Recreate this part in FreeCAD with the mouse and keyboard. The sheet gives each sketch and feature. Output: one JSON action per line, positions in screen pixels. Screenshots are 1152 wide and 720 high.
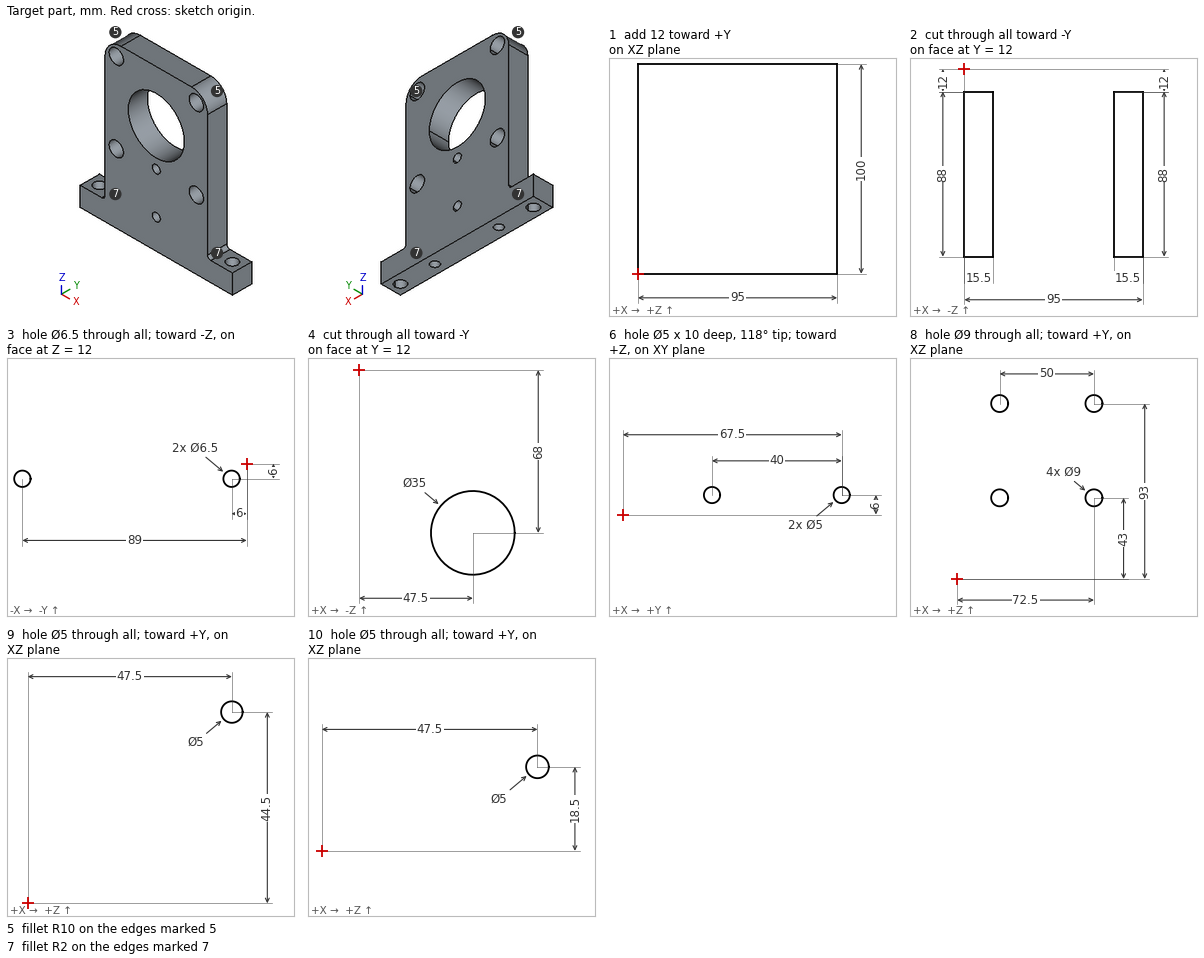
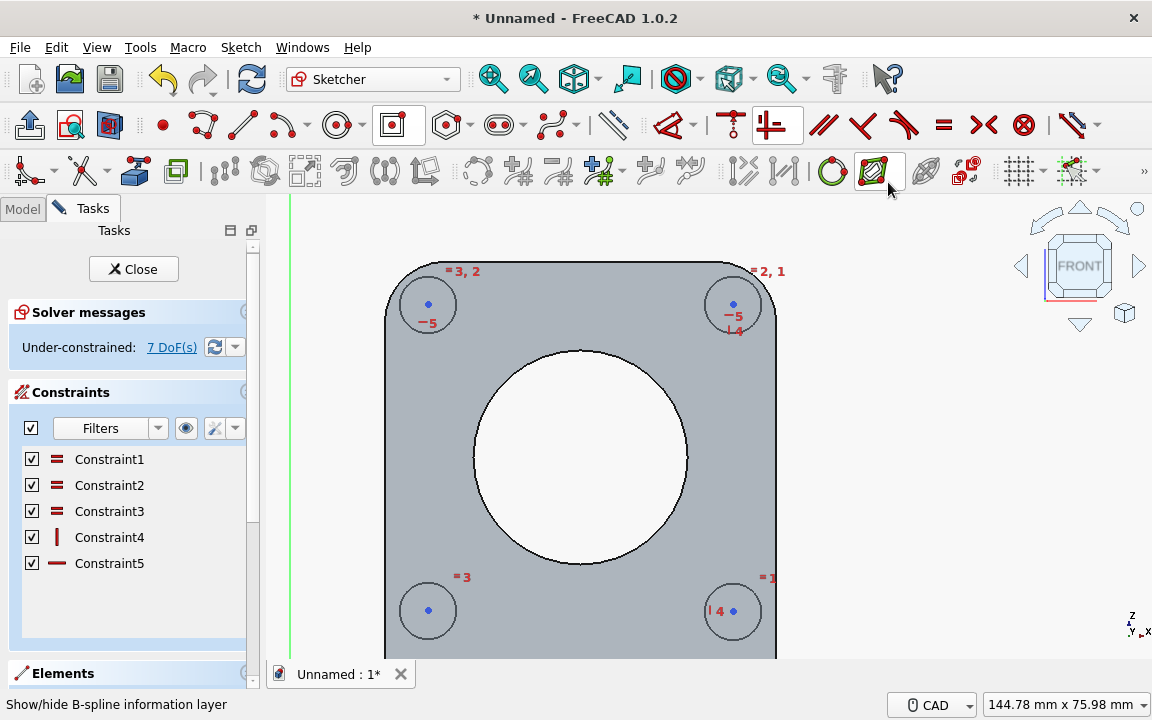
{"action": "left_click", "coordinate": [428, 305]}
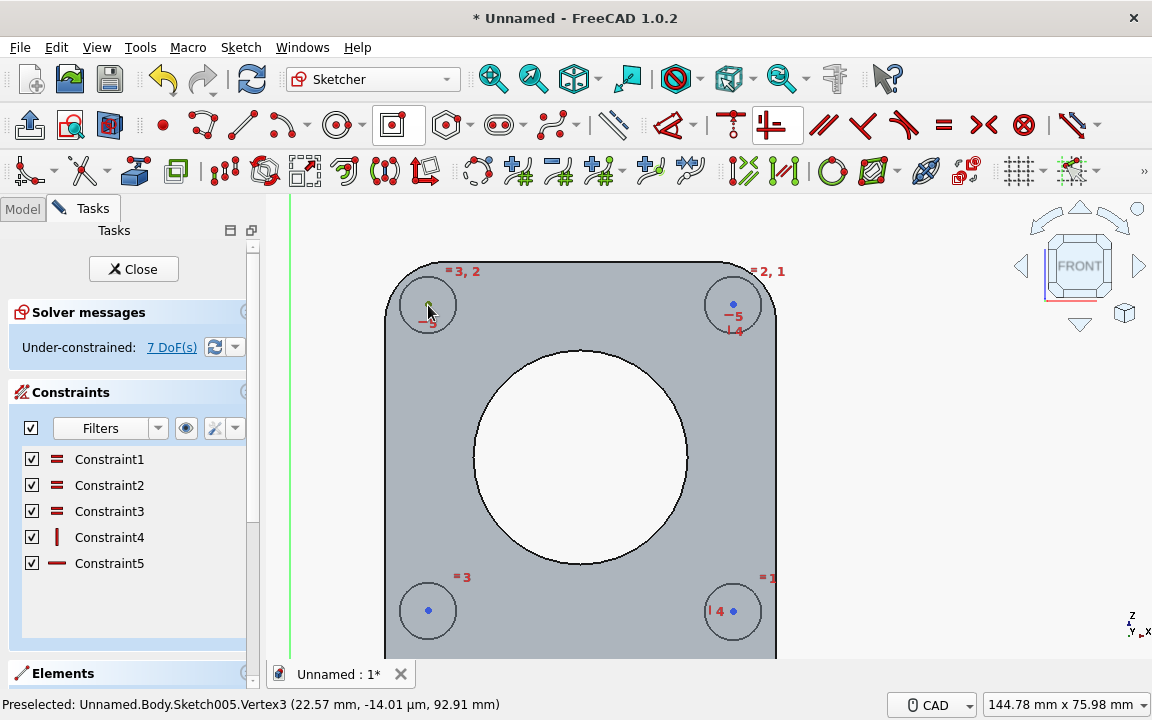
{"action": "left_click", "coordinate": [428, 611]}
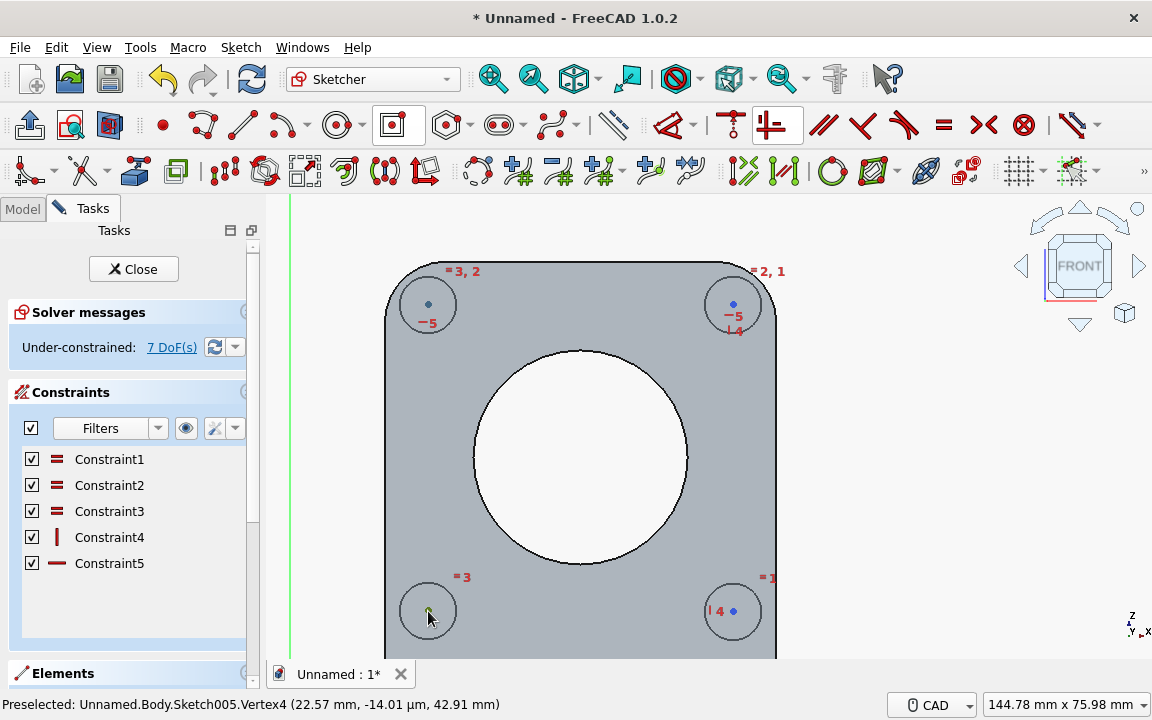
{"action": "left_click", "coordinate": [798, 126]}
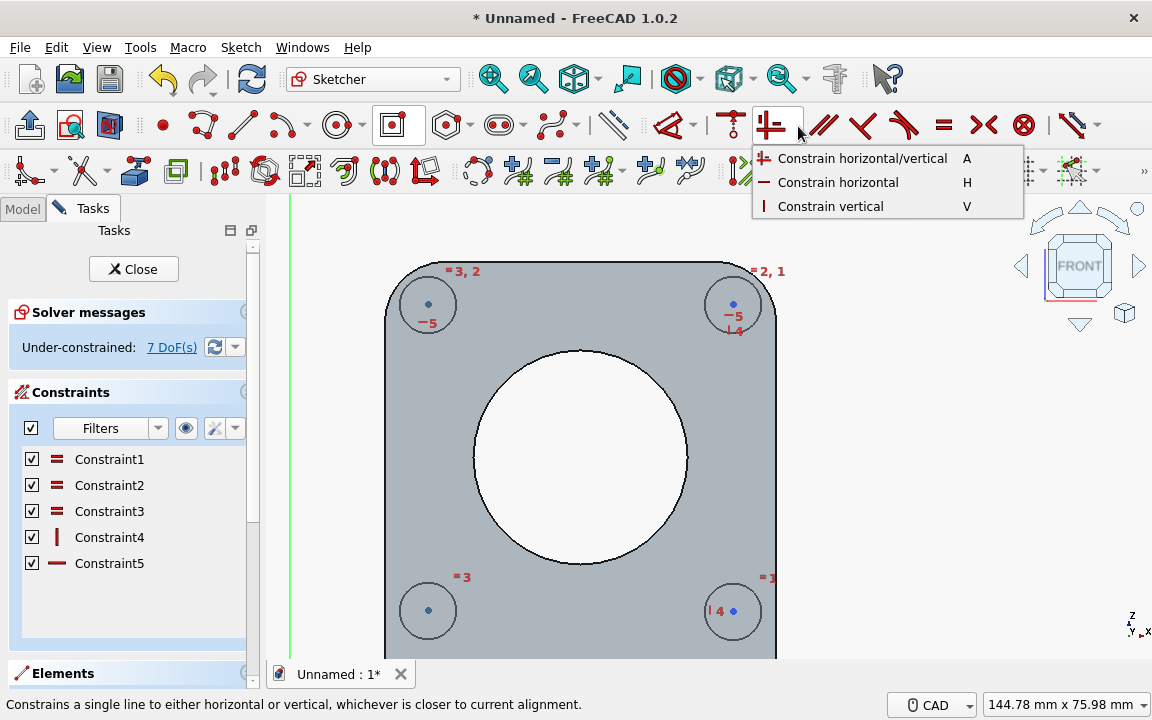
{"action": "left_click", "coordinate": [888, 206]}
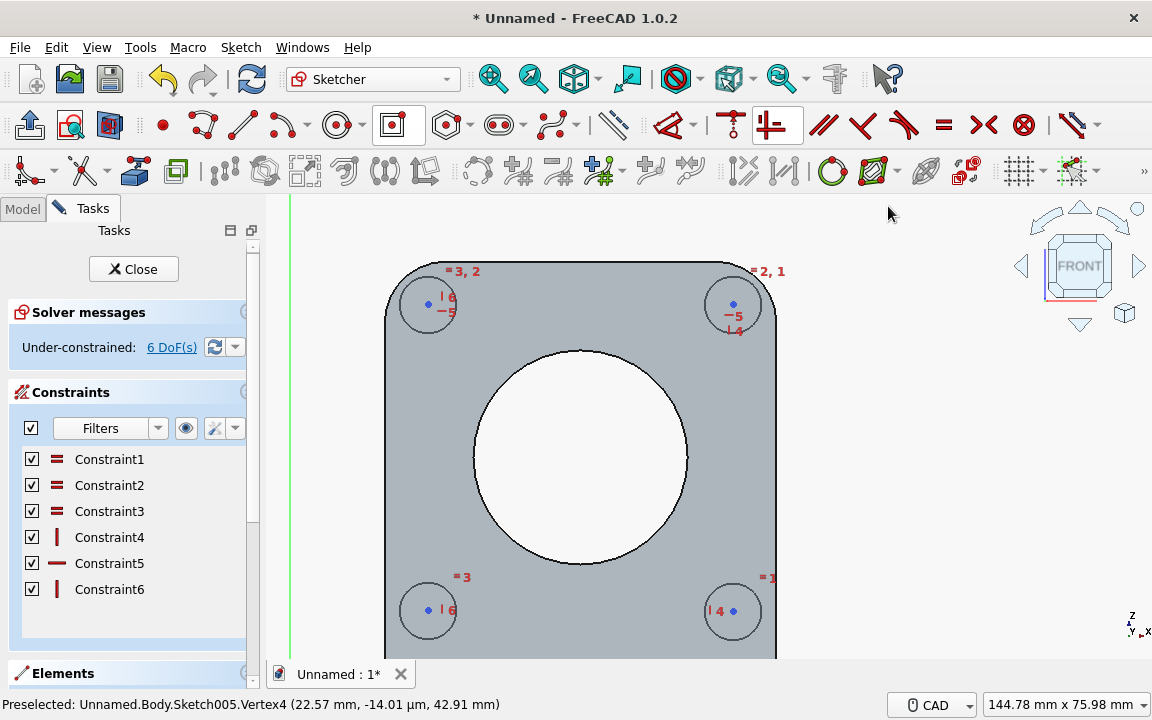
{"action": "left_click", "coordinate": [733, 612]}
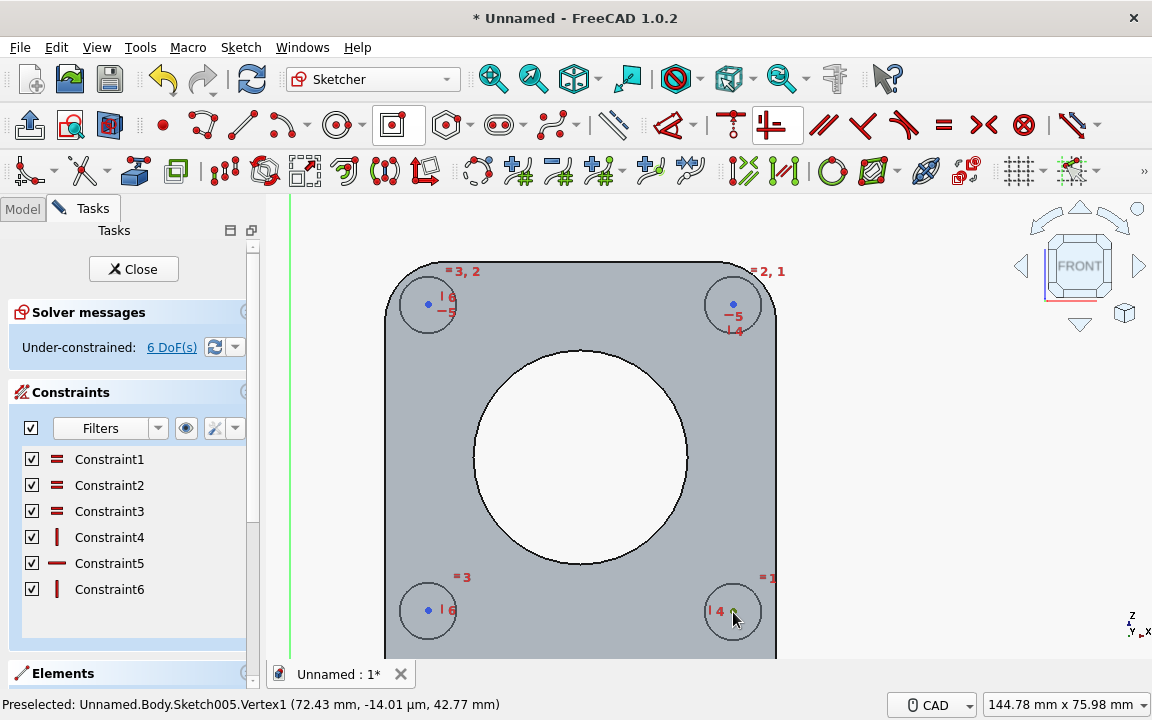
{"action": "left_click", "coordinate": [428, 611]}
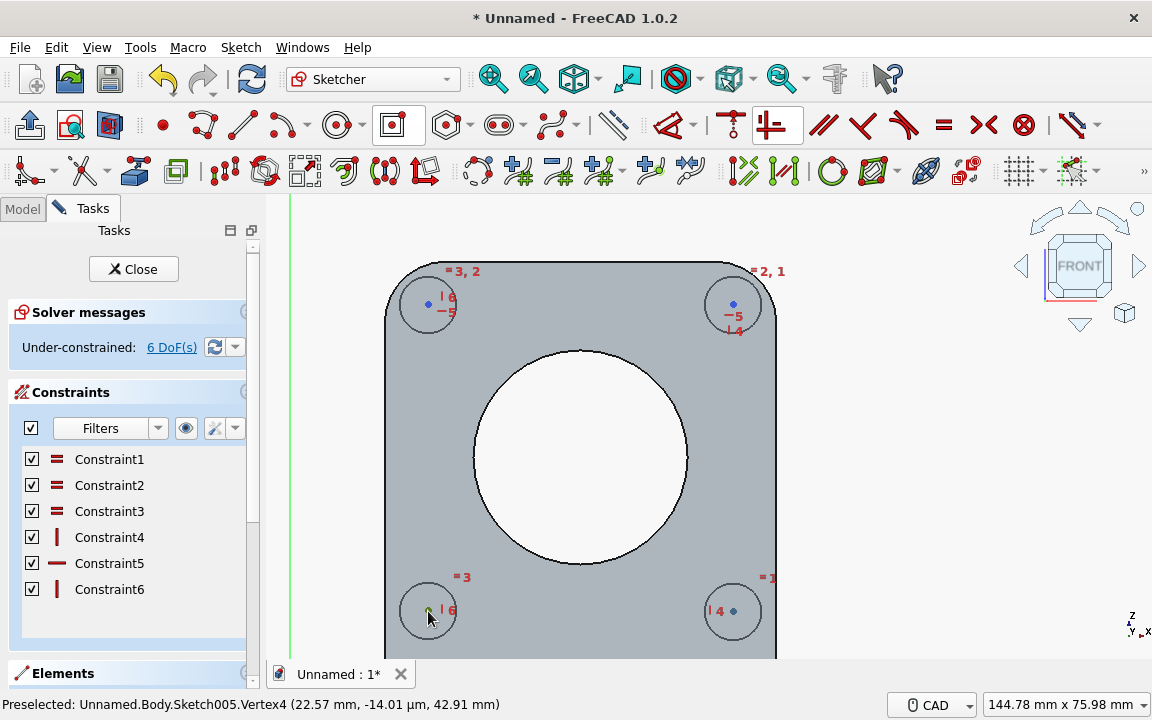
{"action": "left_click", "coordinate": [798, 126]}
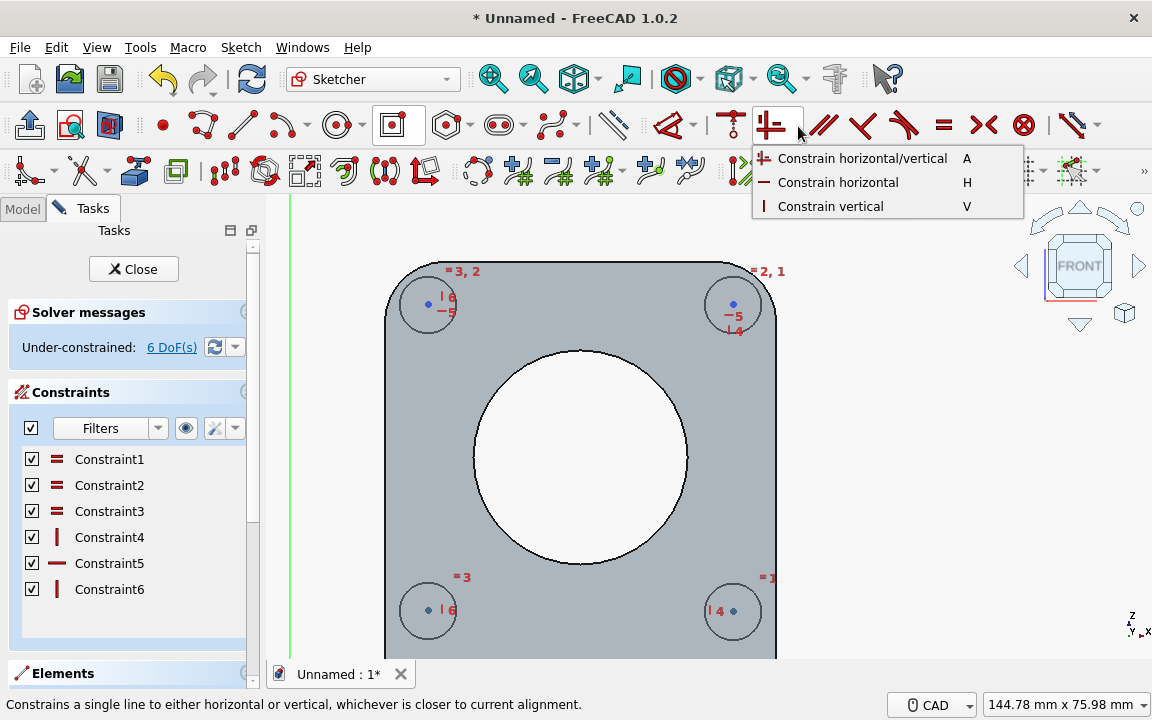
{"action": "left_click", "coordinate": [888, 182]}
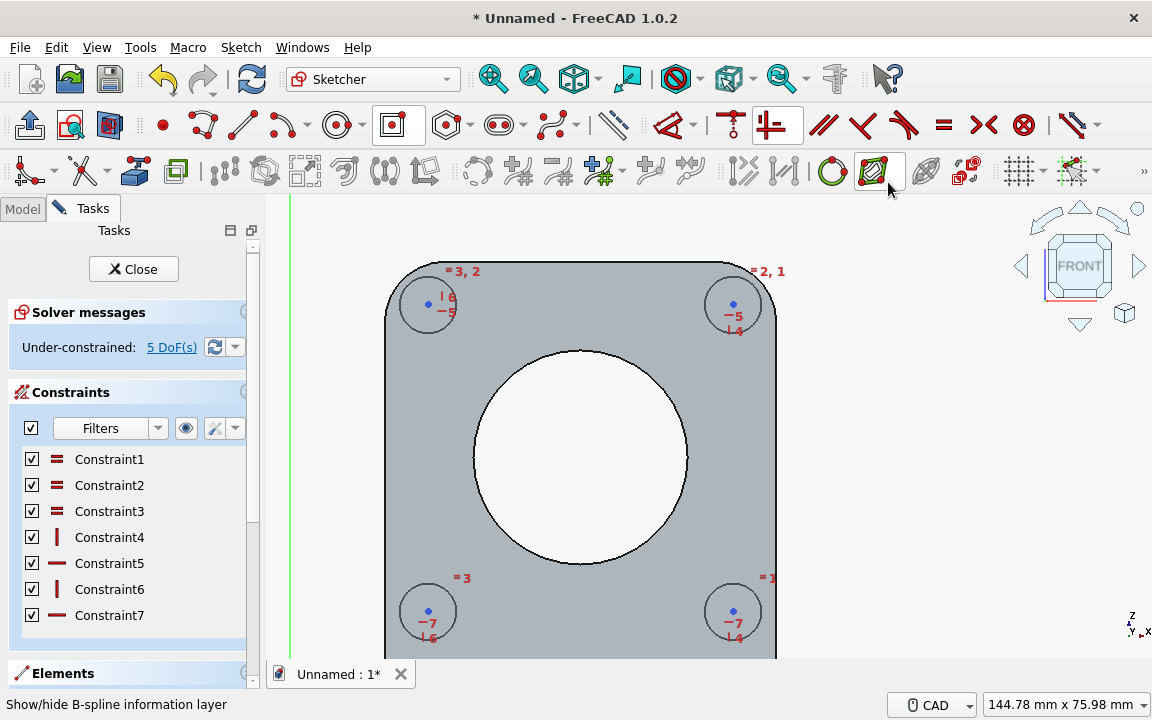
{"action": "left_click", "coordinate": [668, 126]}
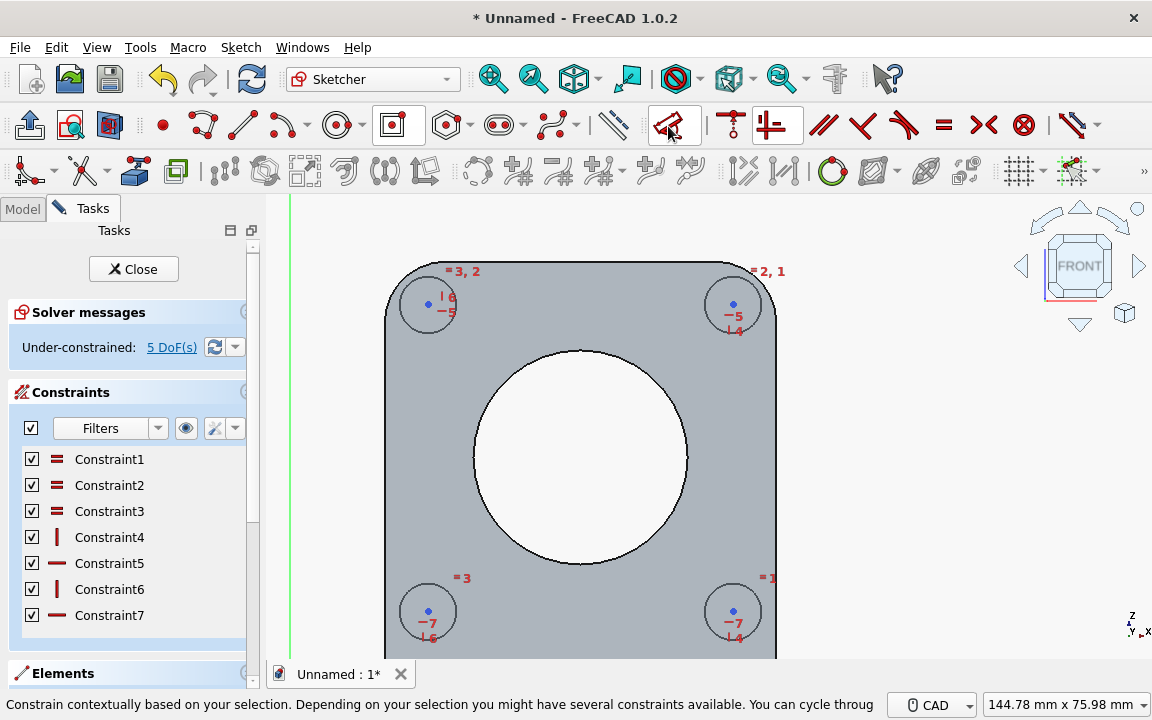
{"action": "left_click", "coordinate": [753, 592]}
{"action": "left_click", "coordinate": [776, 569]}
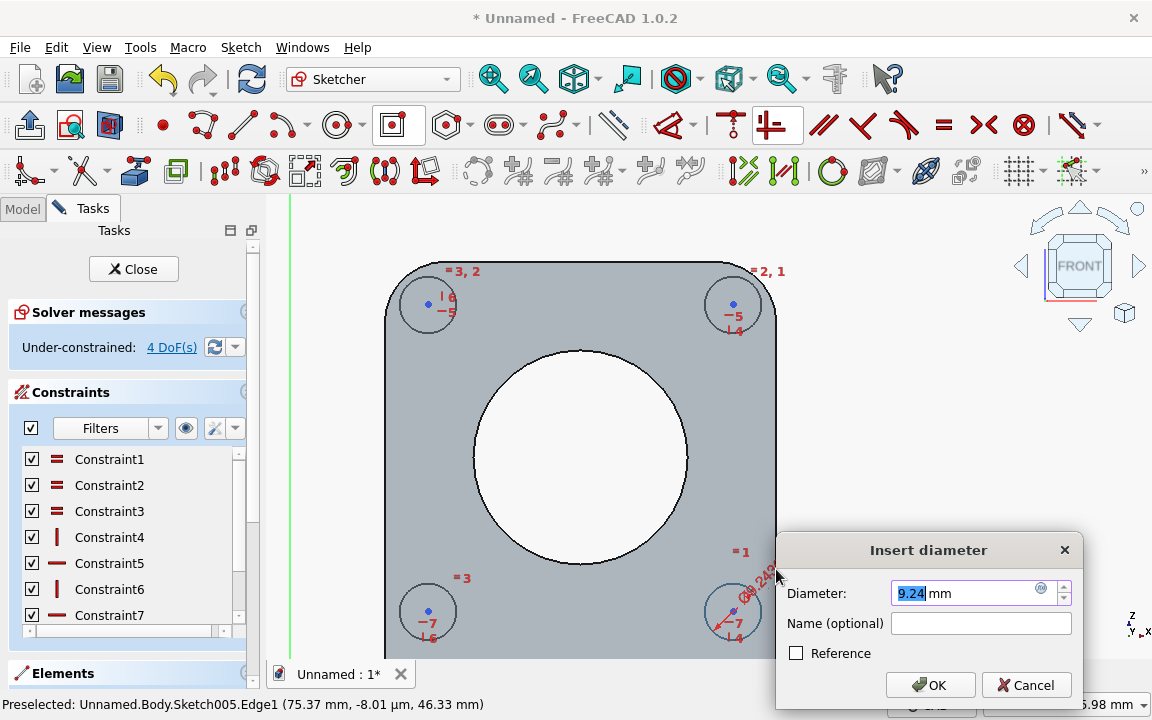
{"action": "type", "text": "9"}
{"action": "key", "text": "Return"}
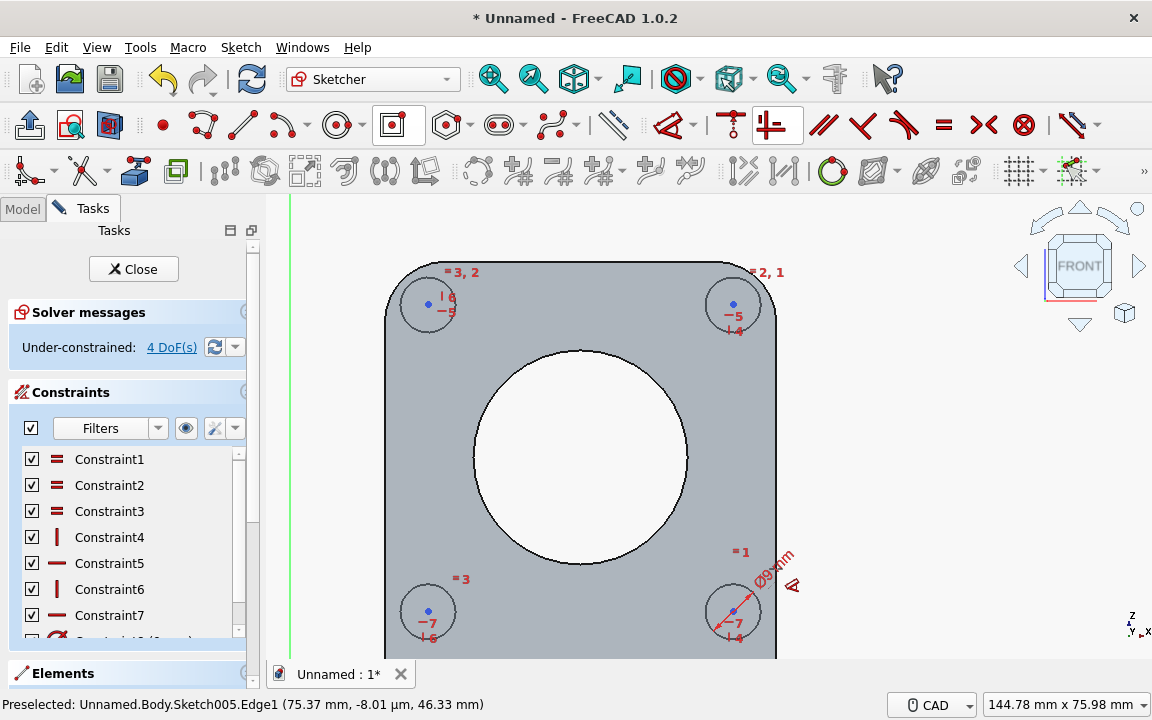
{"action": "left_click", "coordinate": [733, 612]}
{"action": "left_click", "coordinate": [791, 621]}